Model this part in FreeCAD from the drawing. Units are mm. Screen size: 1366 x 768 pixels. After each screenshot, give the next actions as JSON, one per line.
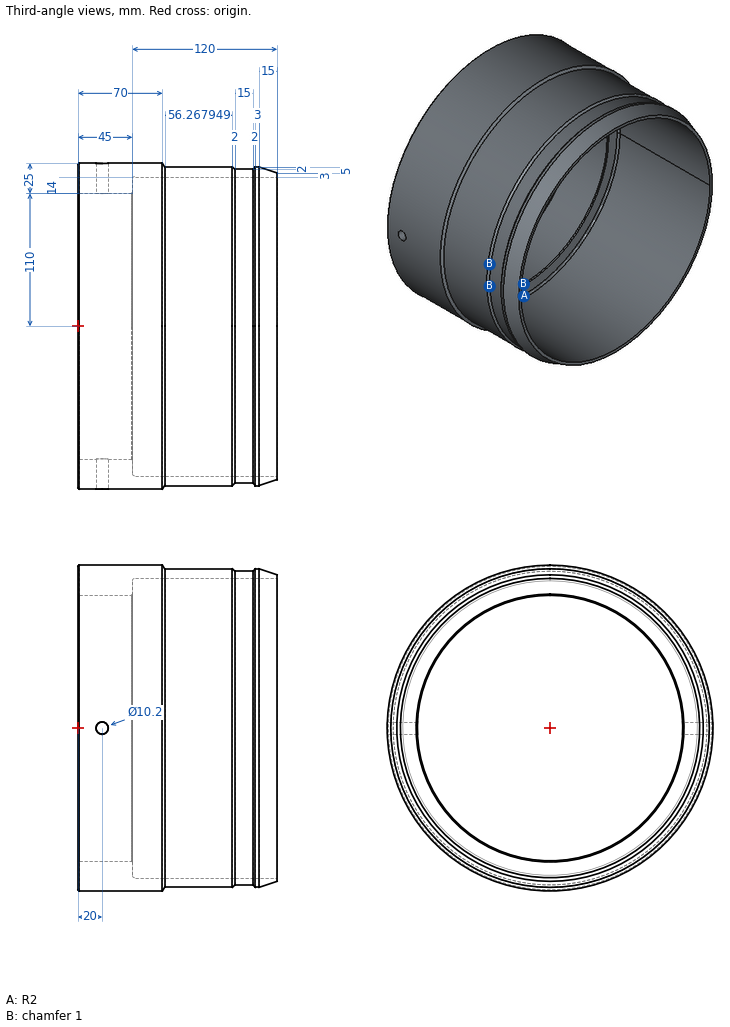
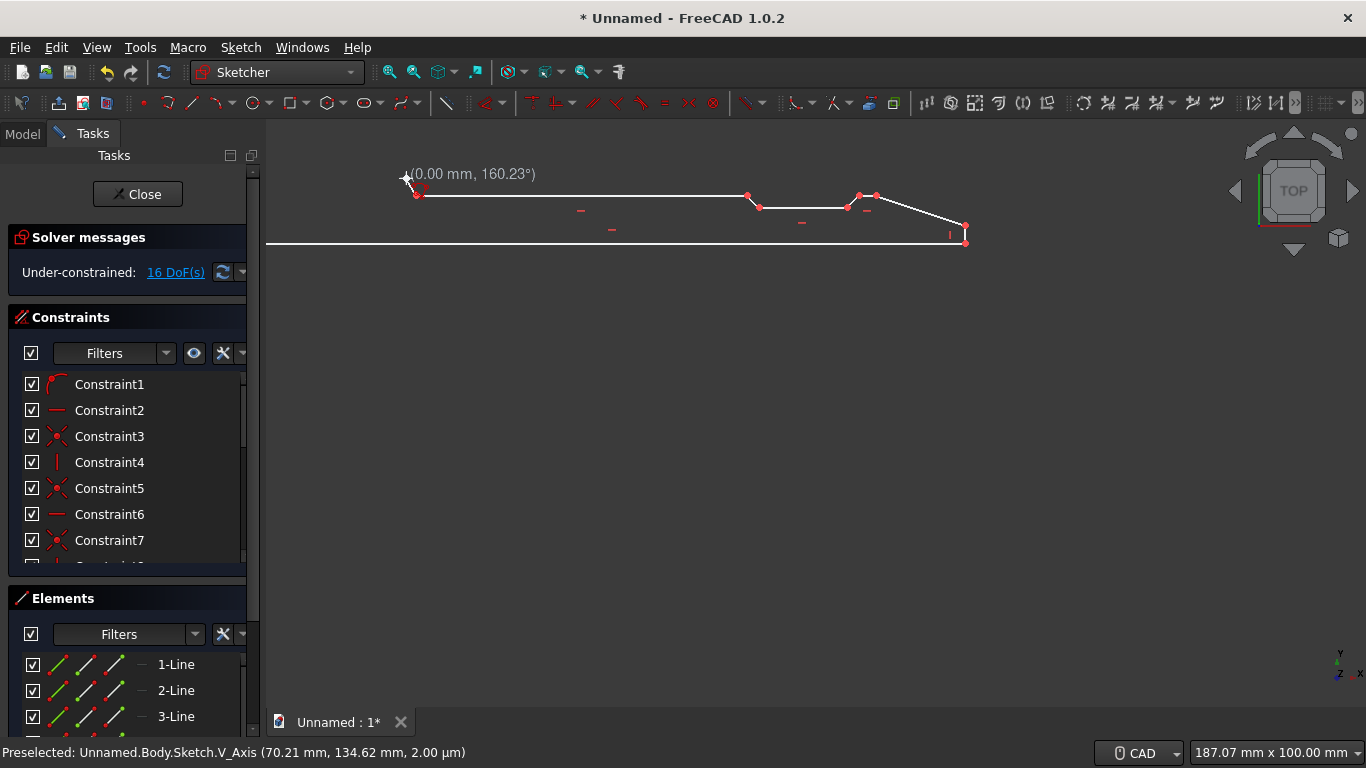
{"action": "scroll", "coordinate": [966, 281], "scroll_direction": "down", "scroll_amount": 4}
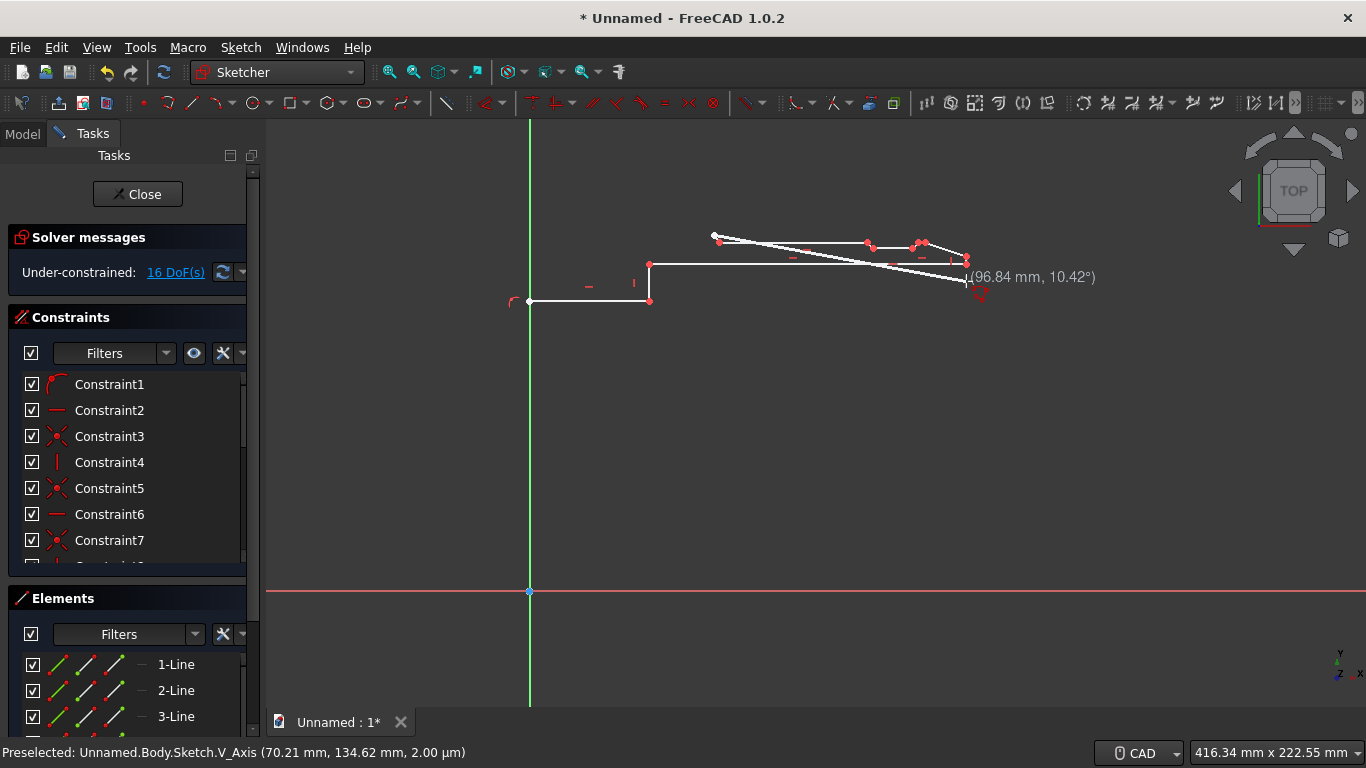
{"action": "left_click", "coordinate": [539, 235]}
{"action": "left_click", "coordinate": [530, 301]}
{"action": "key", "text": "Escape"}
{"action": "key", "text": "Escape"}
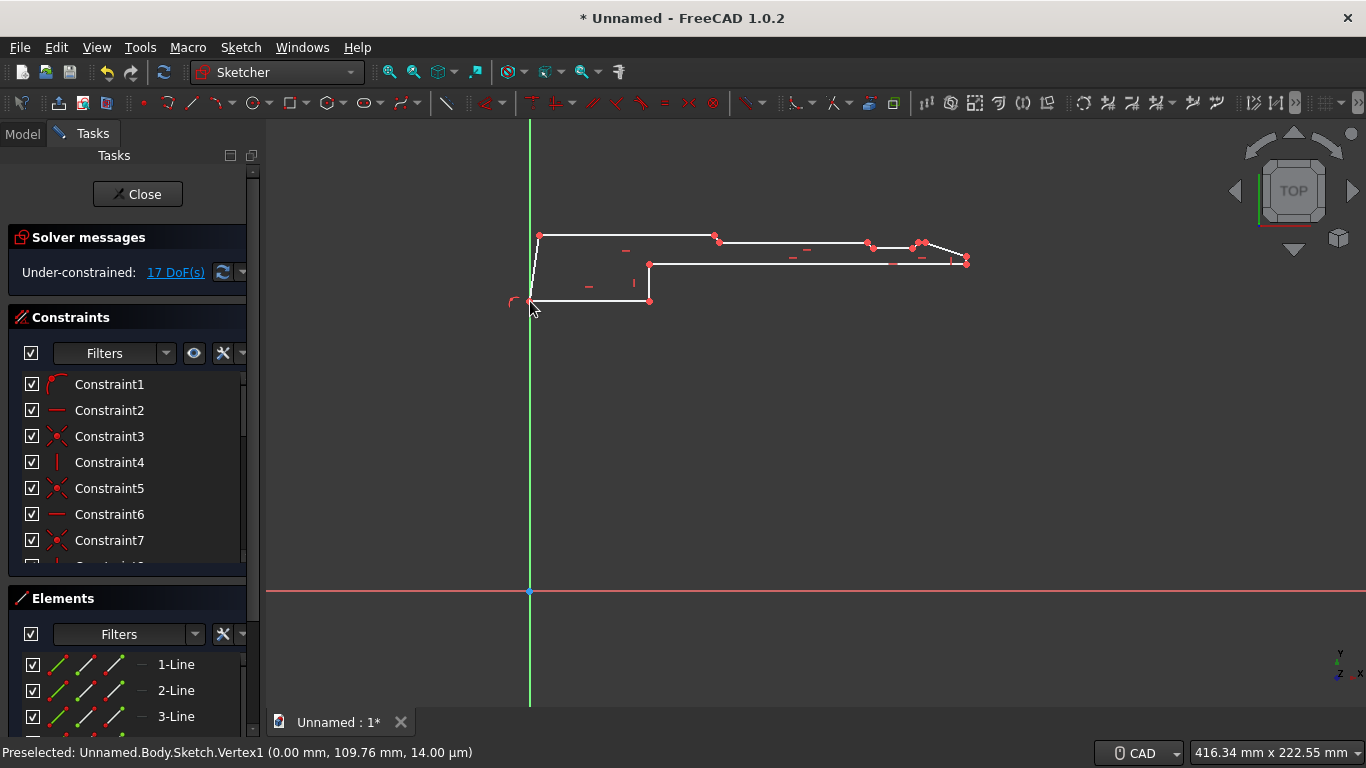
{"action": "left_click", "coordinate": [532, 282]}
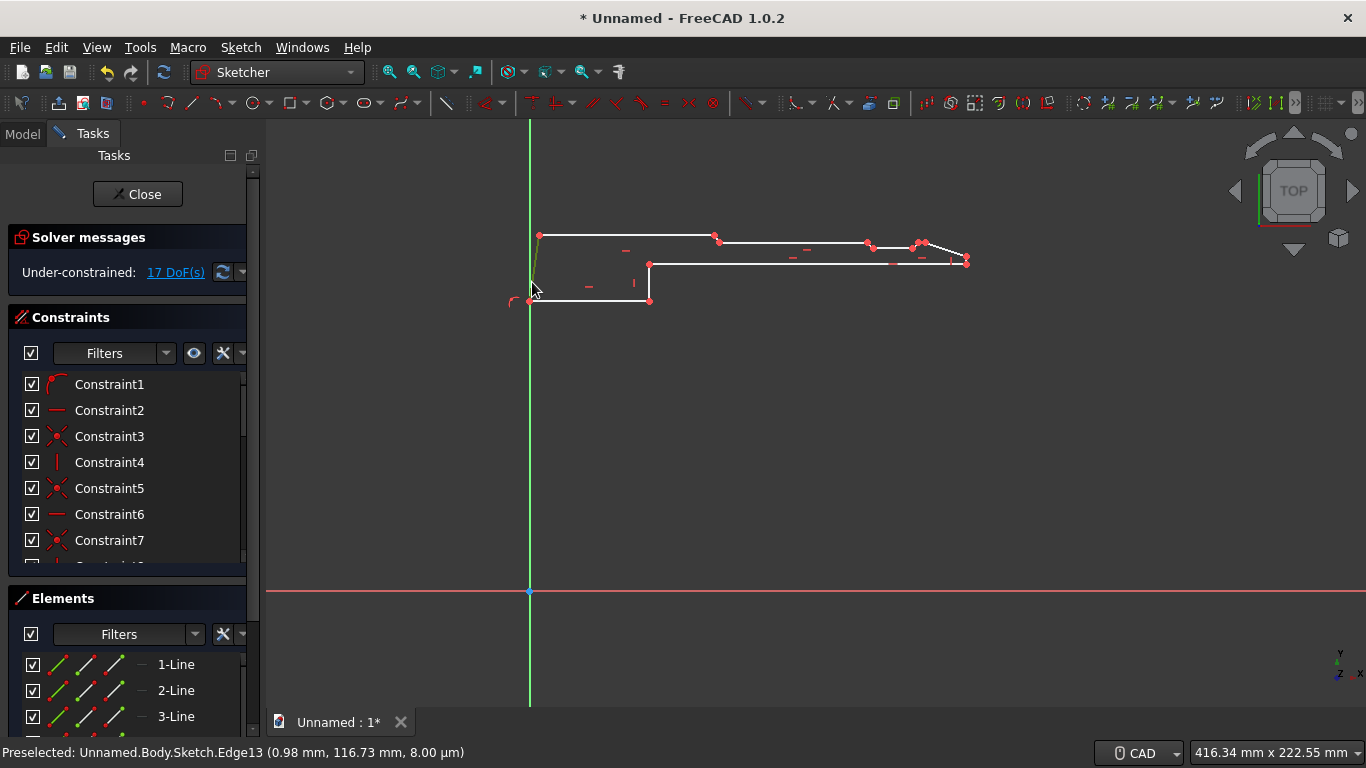
{"action": "key", "text": "v"}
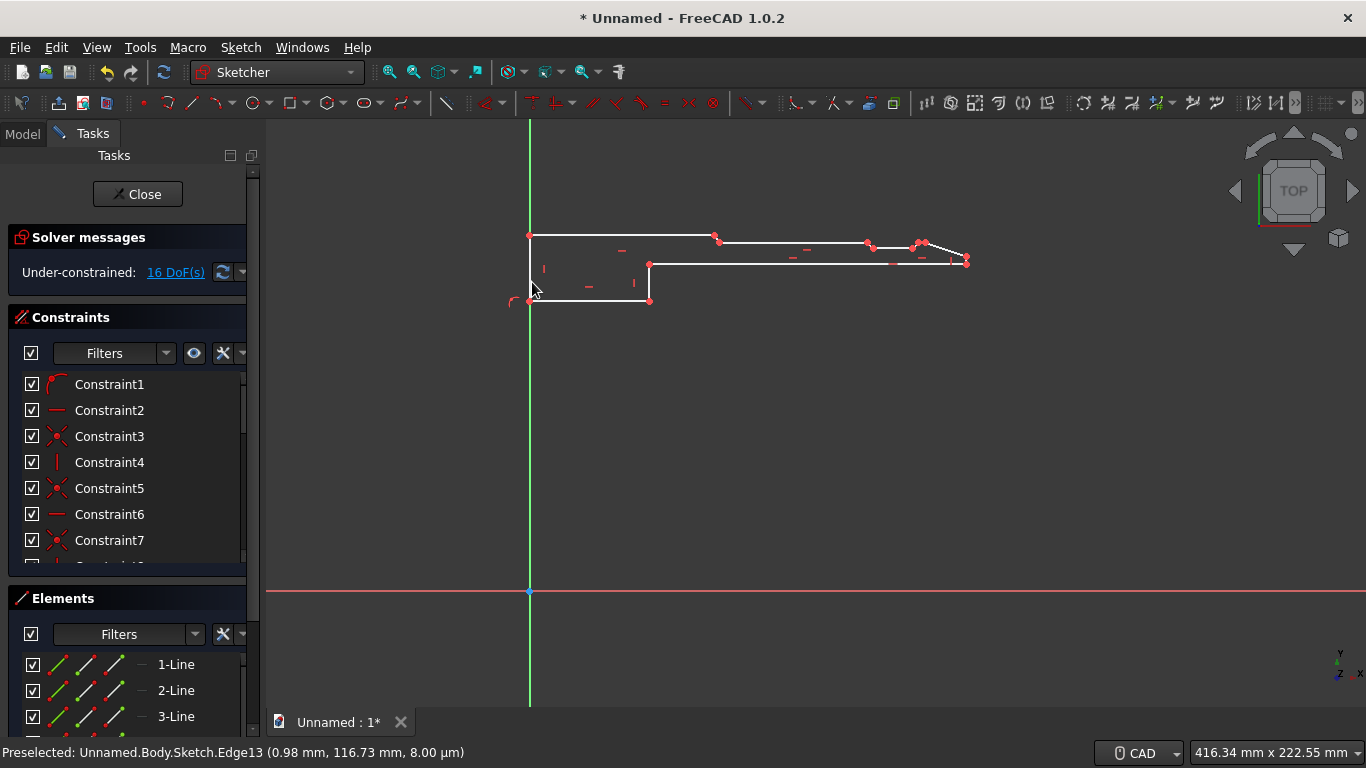
{"action": "left_click", "coordinate": [486, 104]}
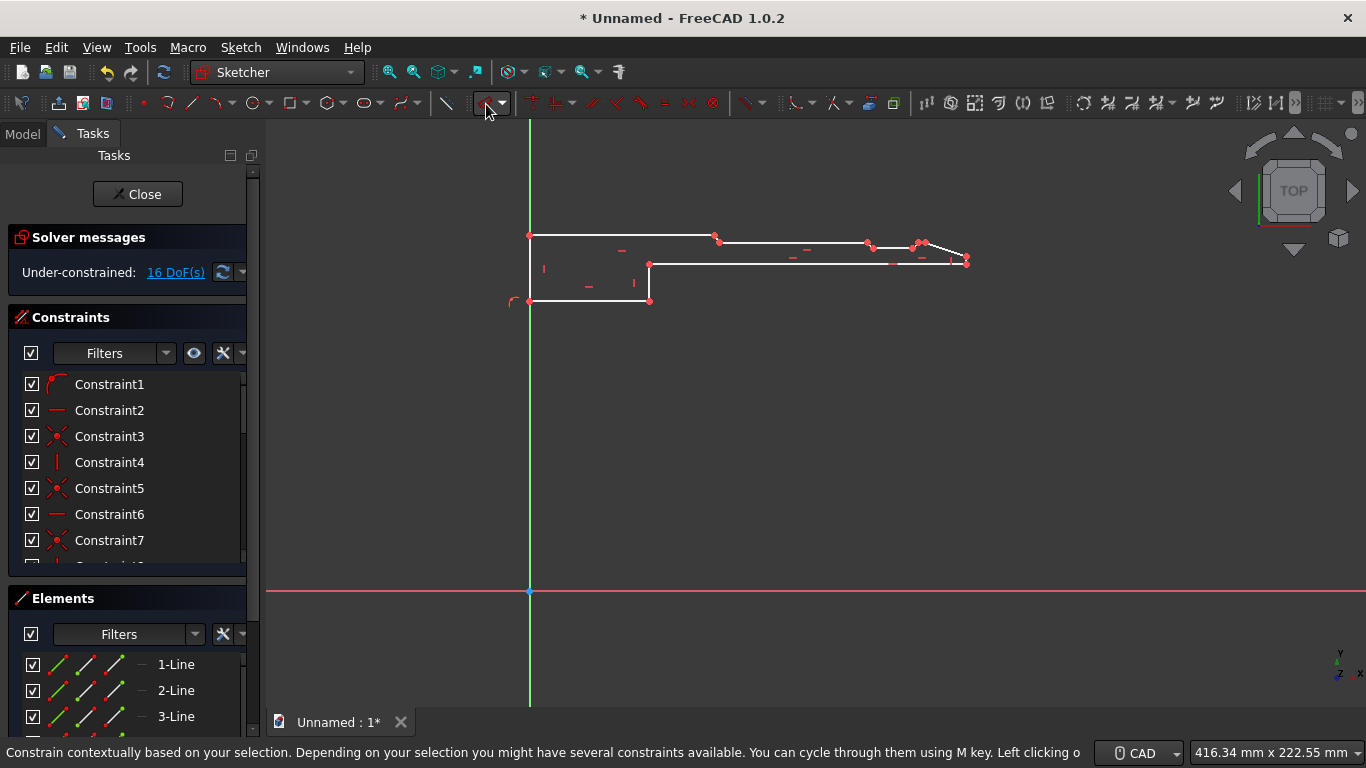
{"action": "scroll", "coordinate": [966, 260], "scroll_direction": "up", "scroll_amount": 9}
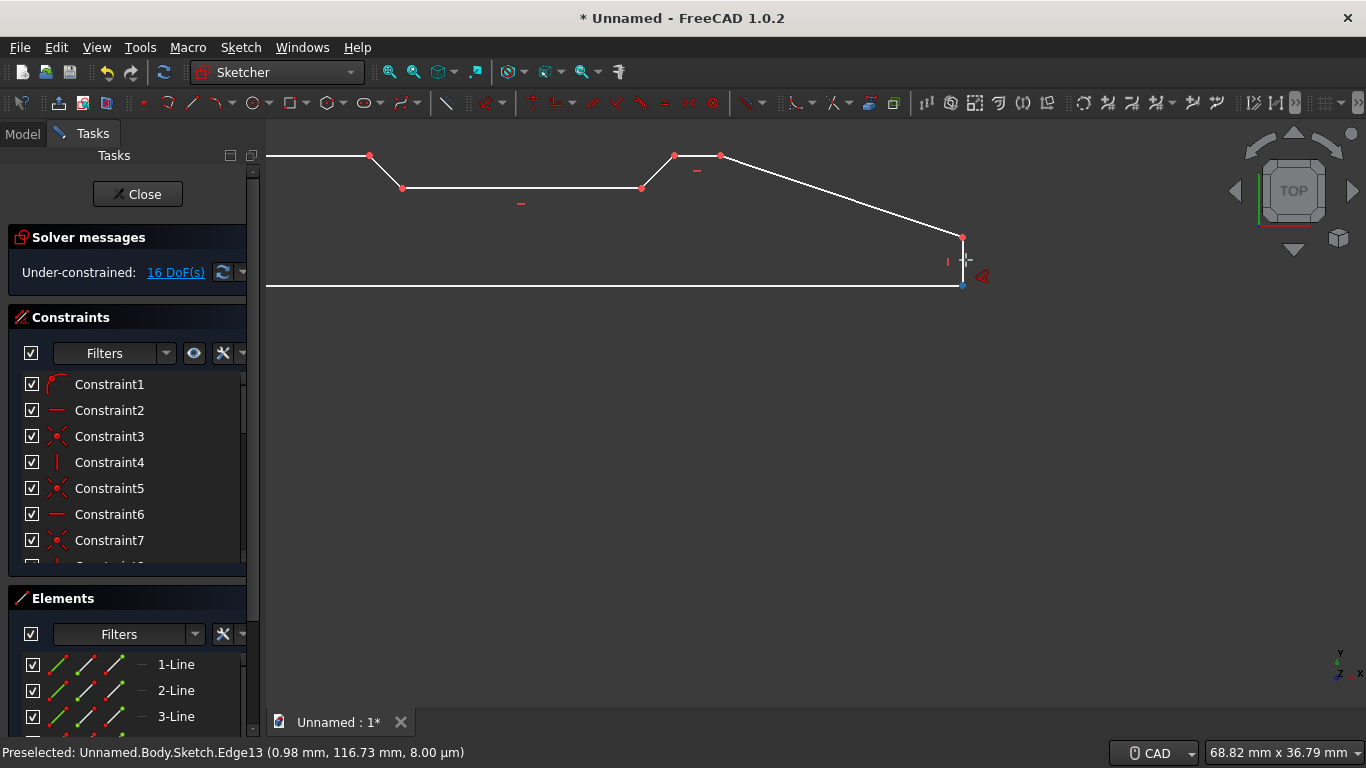
{"action": "left_click", "coordinate": [963, 261]}
{"action": "left_click", "coordinate": [997, 261]}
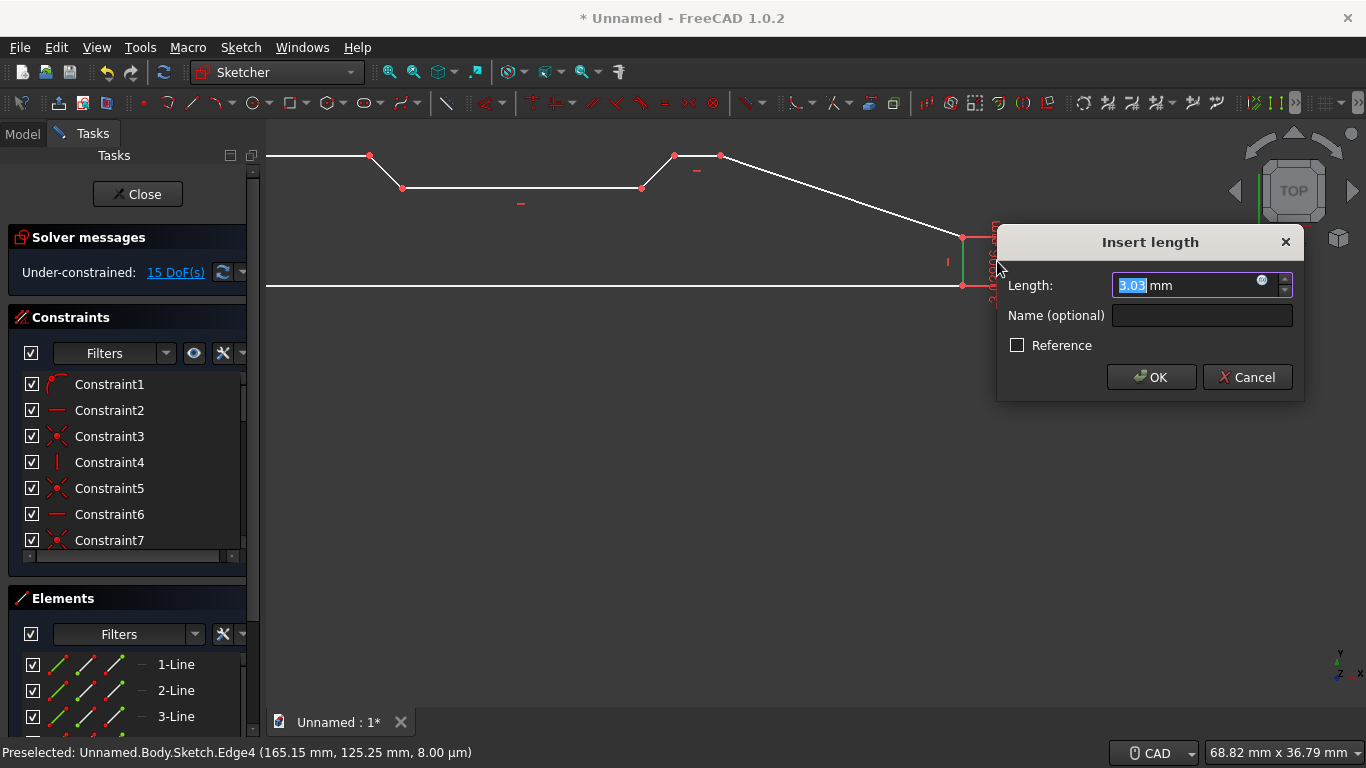
{"action": "type", "text": "3"}
{"action": "key", "text": "Return"}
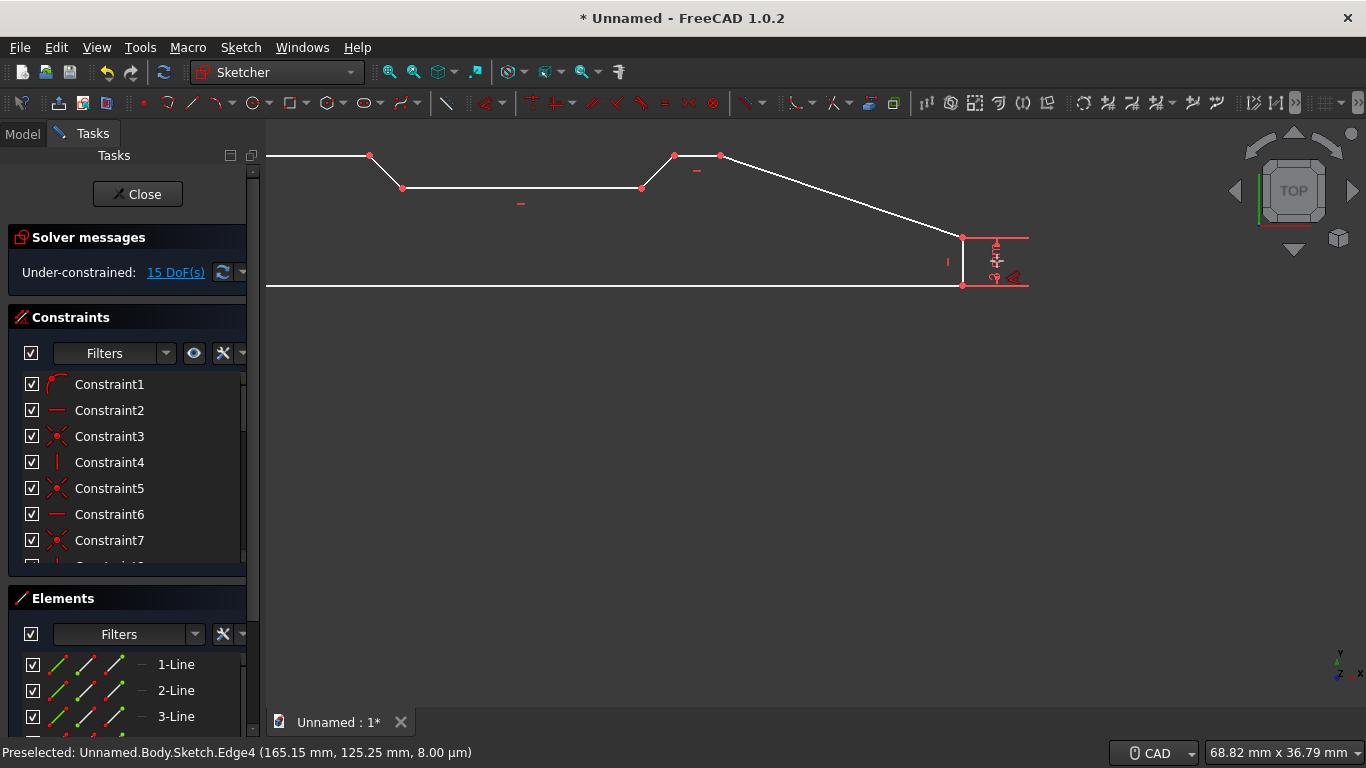
{"action": "left_click", "coordinate": [706, 156]}
{"action": "left_click", "coordinate": [697, 190]}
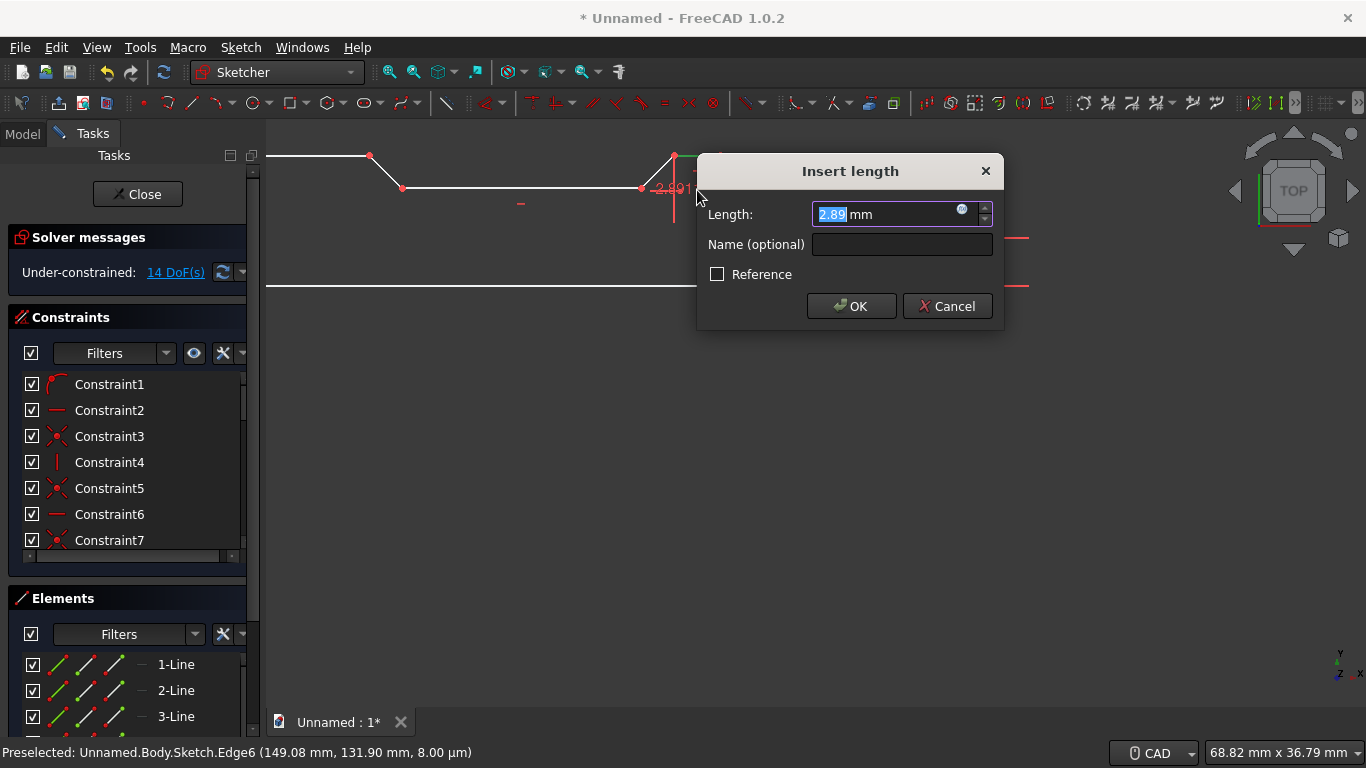
{"action": "type", "text": "3"}
{"action": "key", "text": "Return"}